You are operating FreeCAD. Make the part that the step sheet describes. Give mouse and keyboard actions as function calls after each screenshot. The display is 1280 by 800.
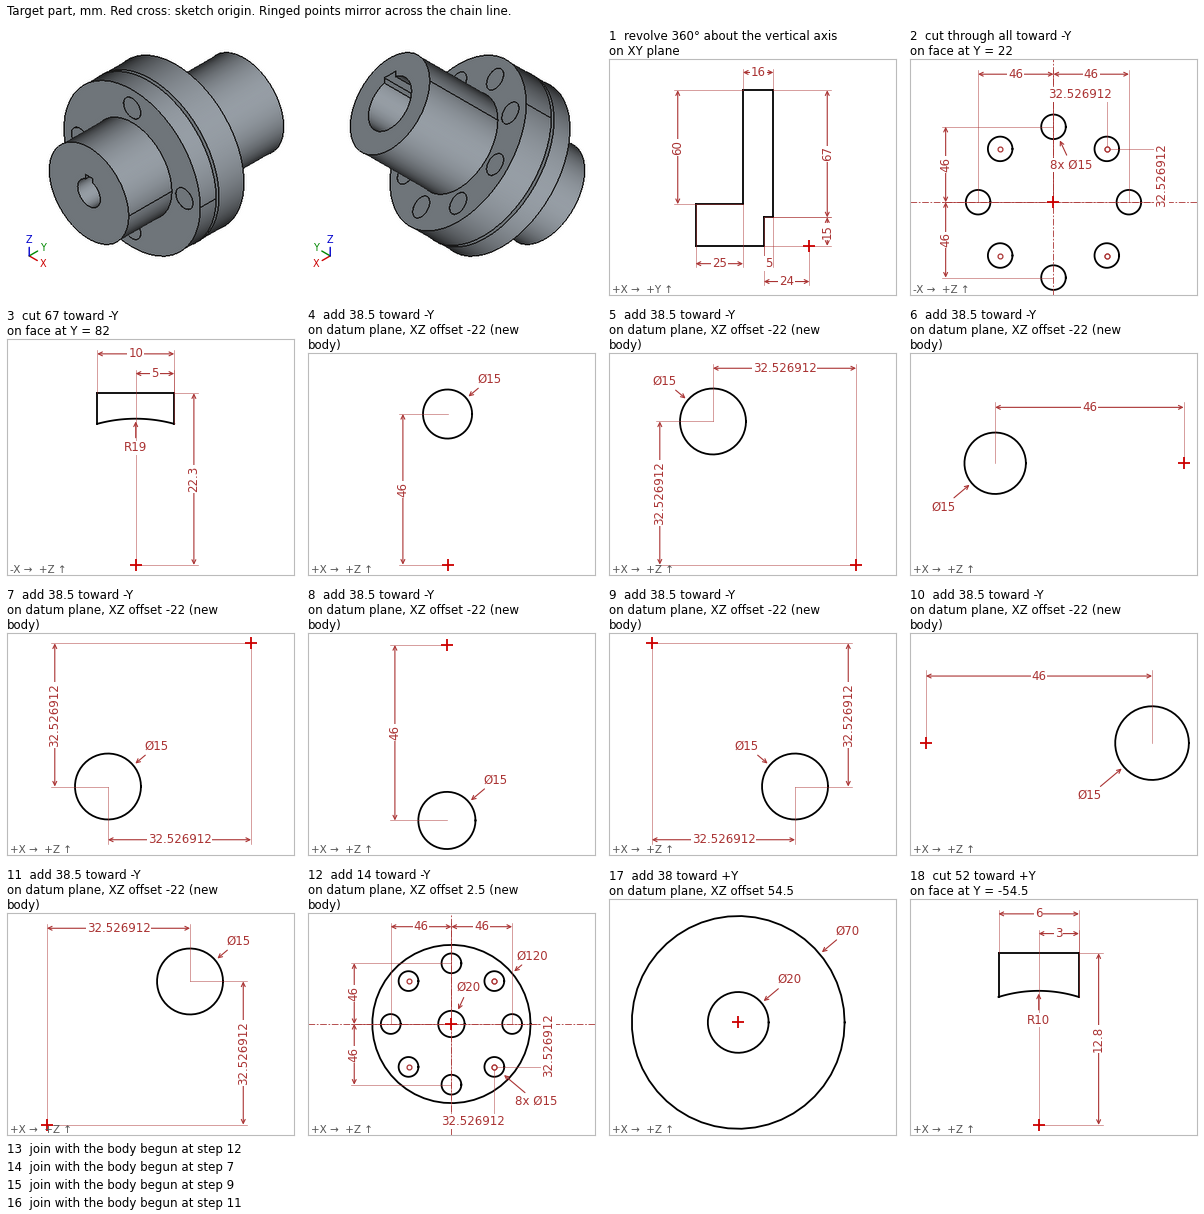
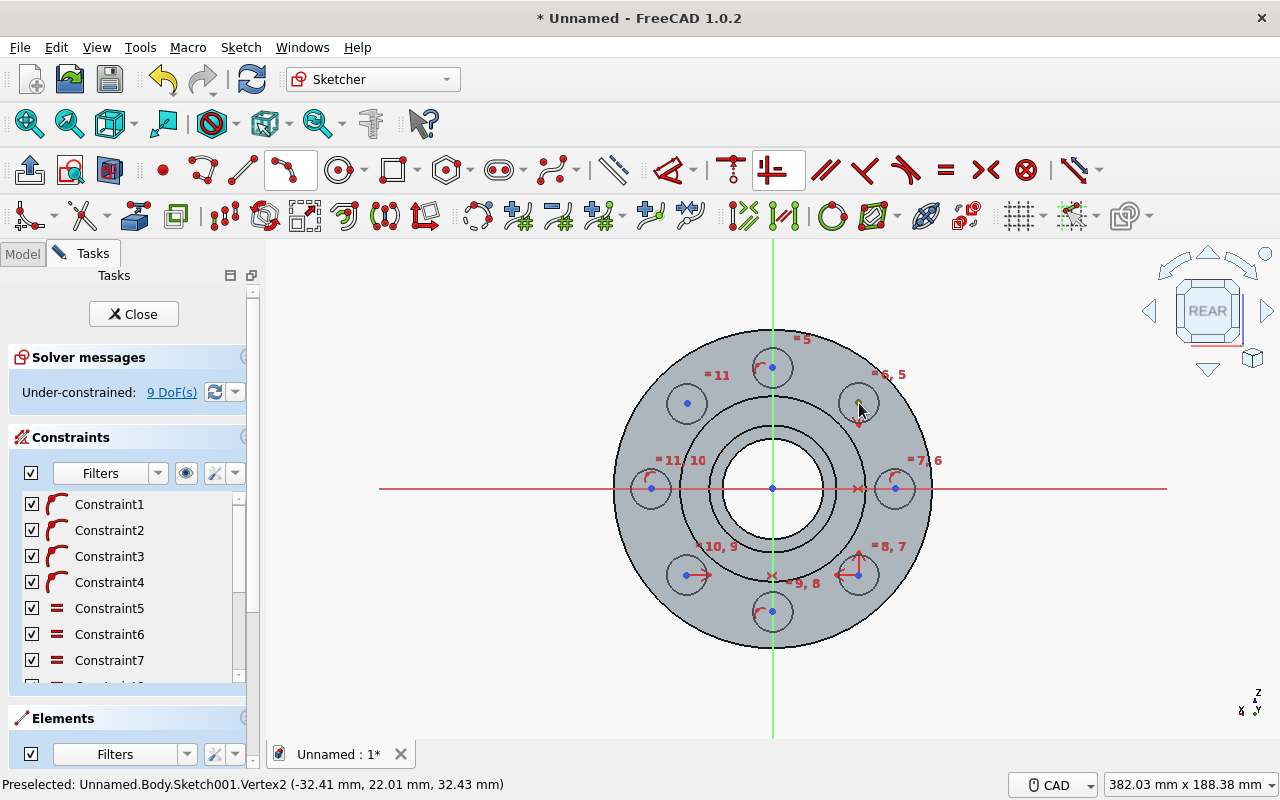
click(687, 404)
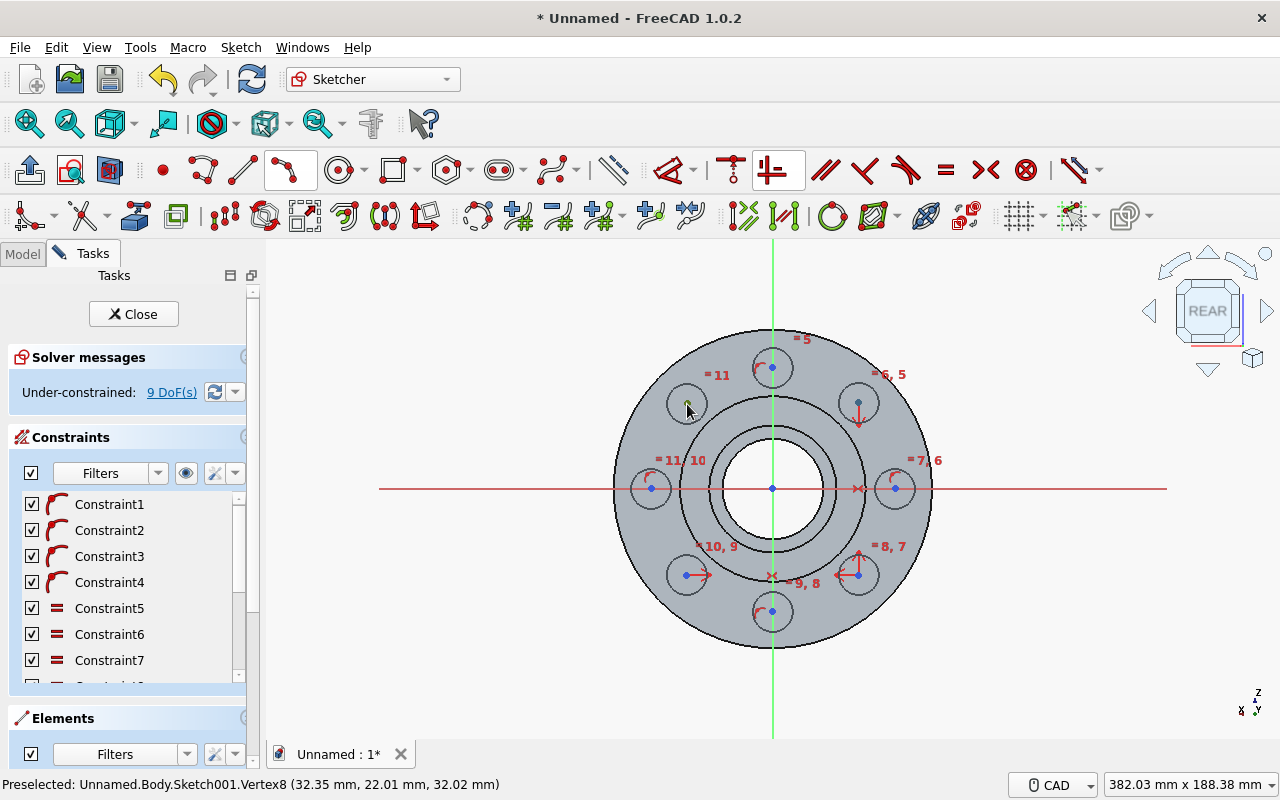
click(773, 679)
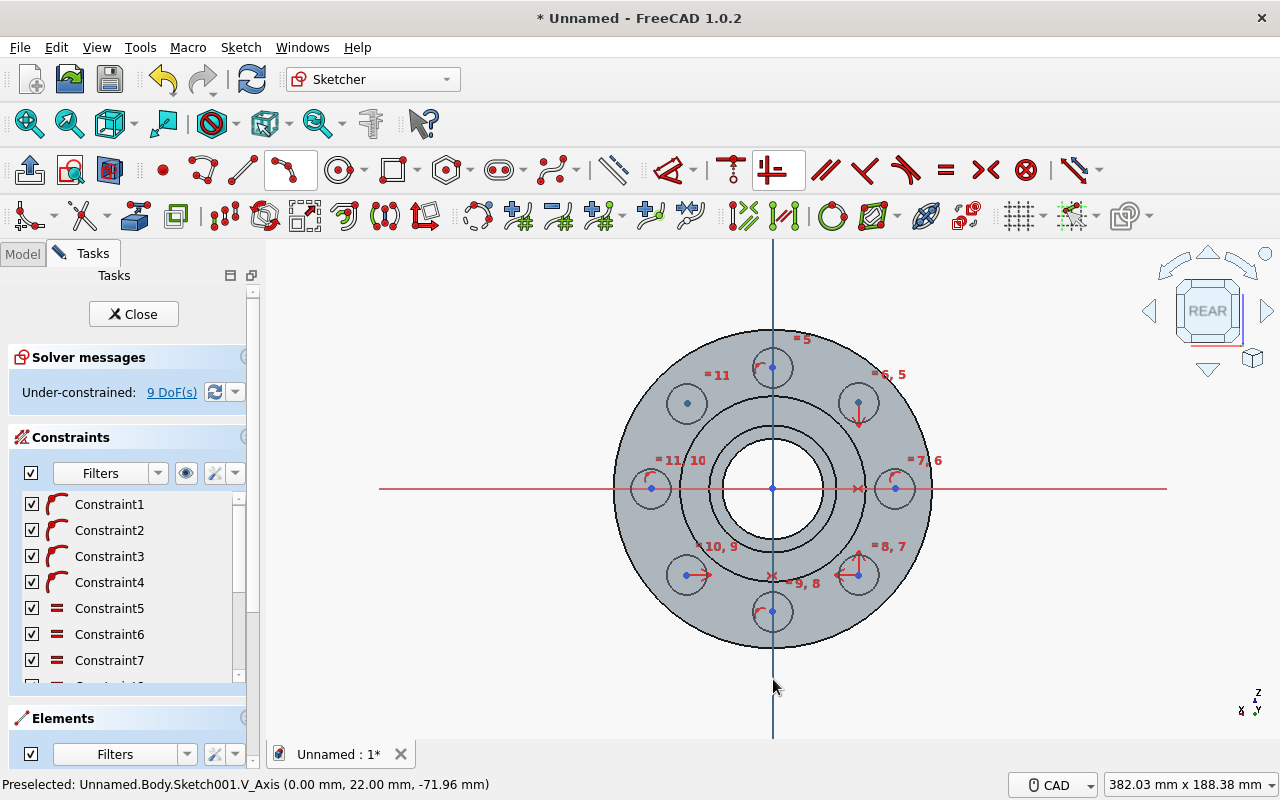
click(986, 170)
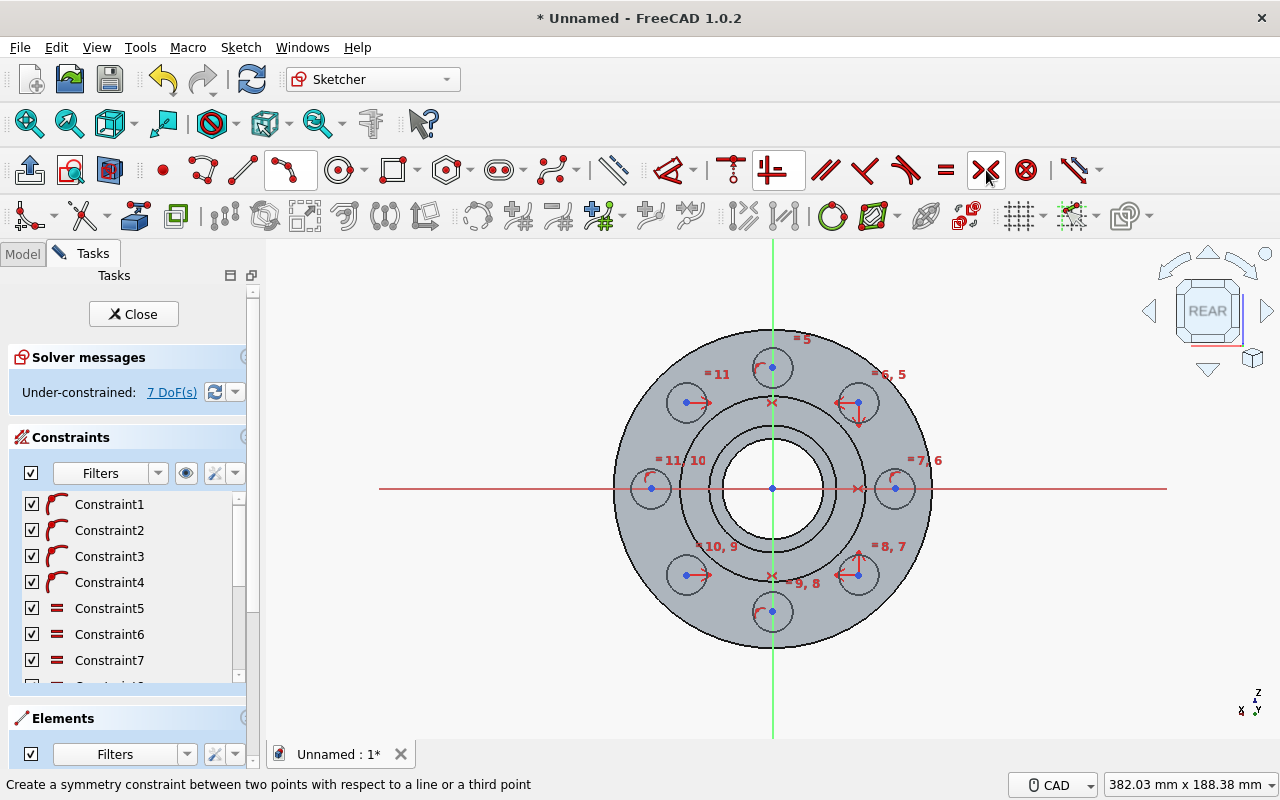
click(668, 170)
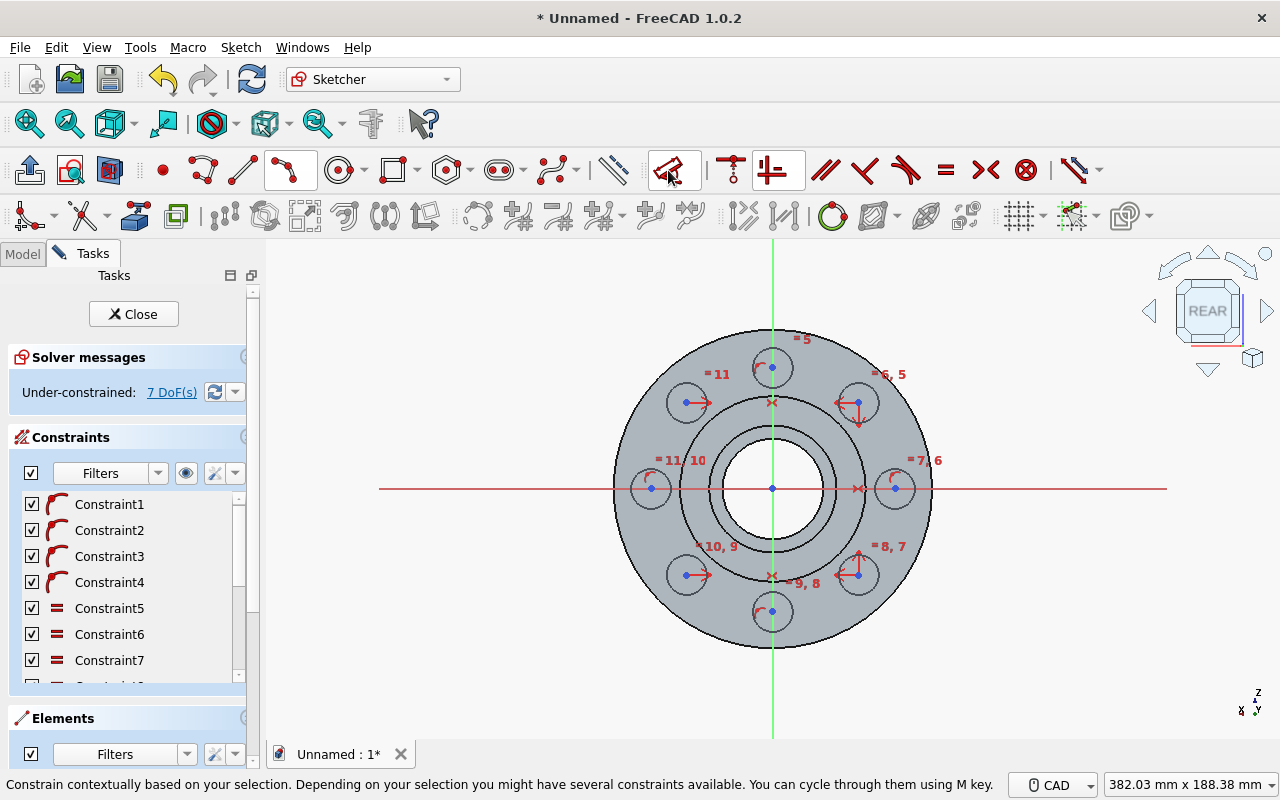
click(787, 354)
click(810, 331)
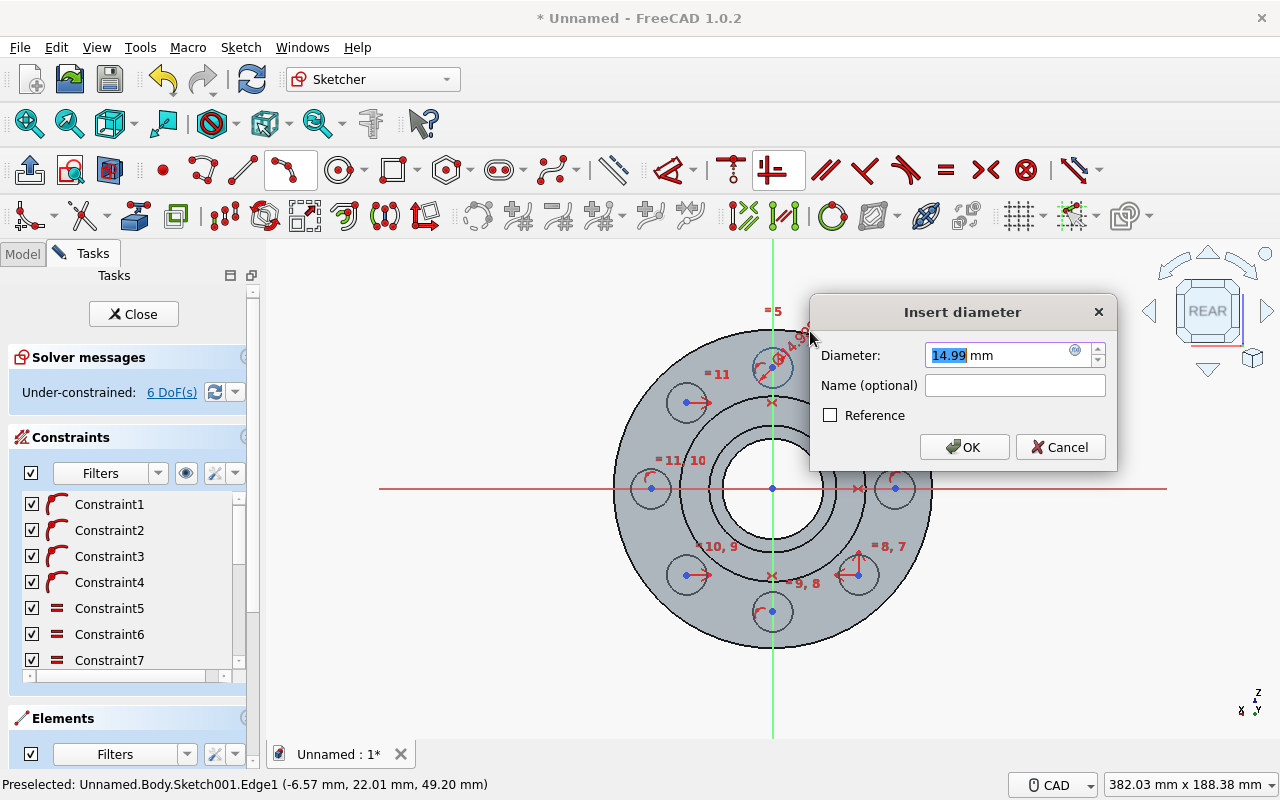
text(15)
key(Return)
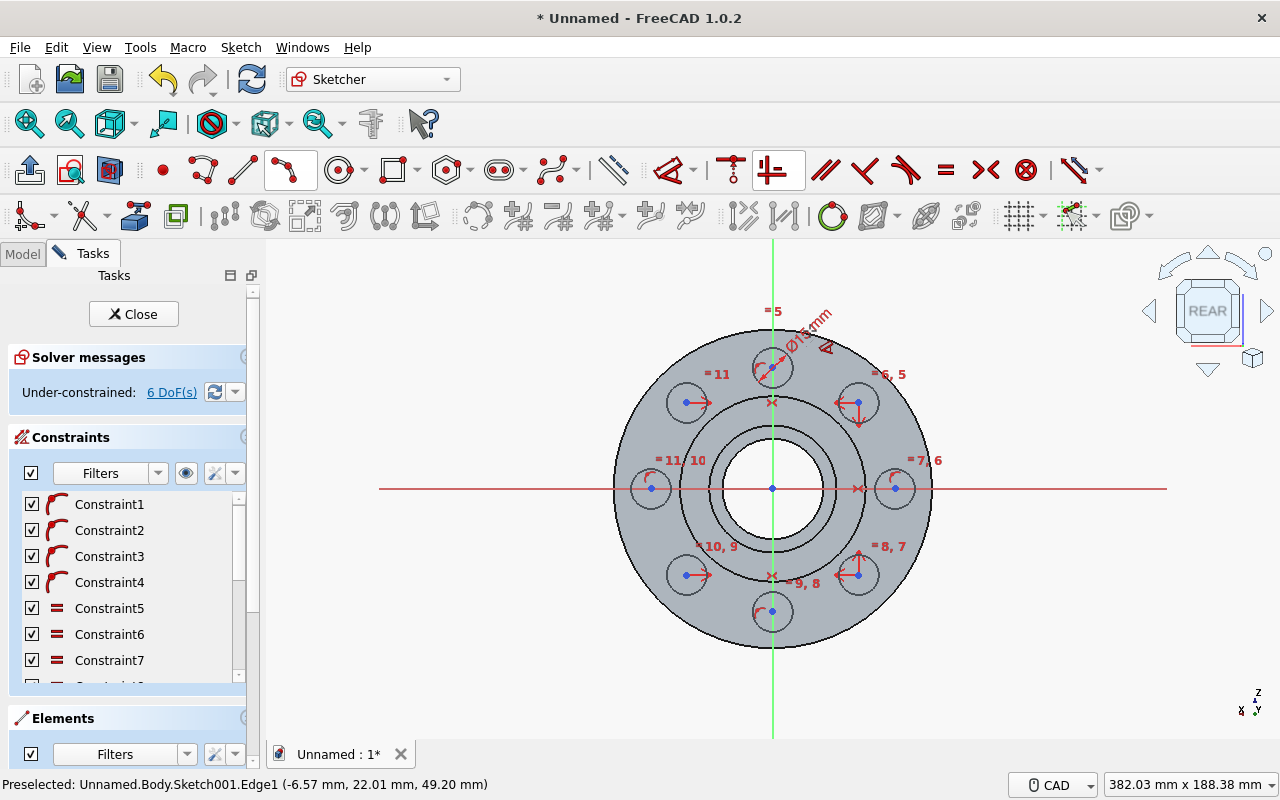
click(773, 368)
click(807, 428)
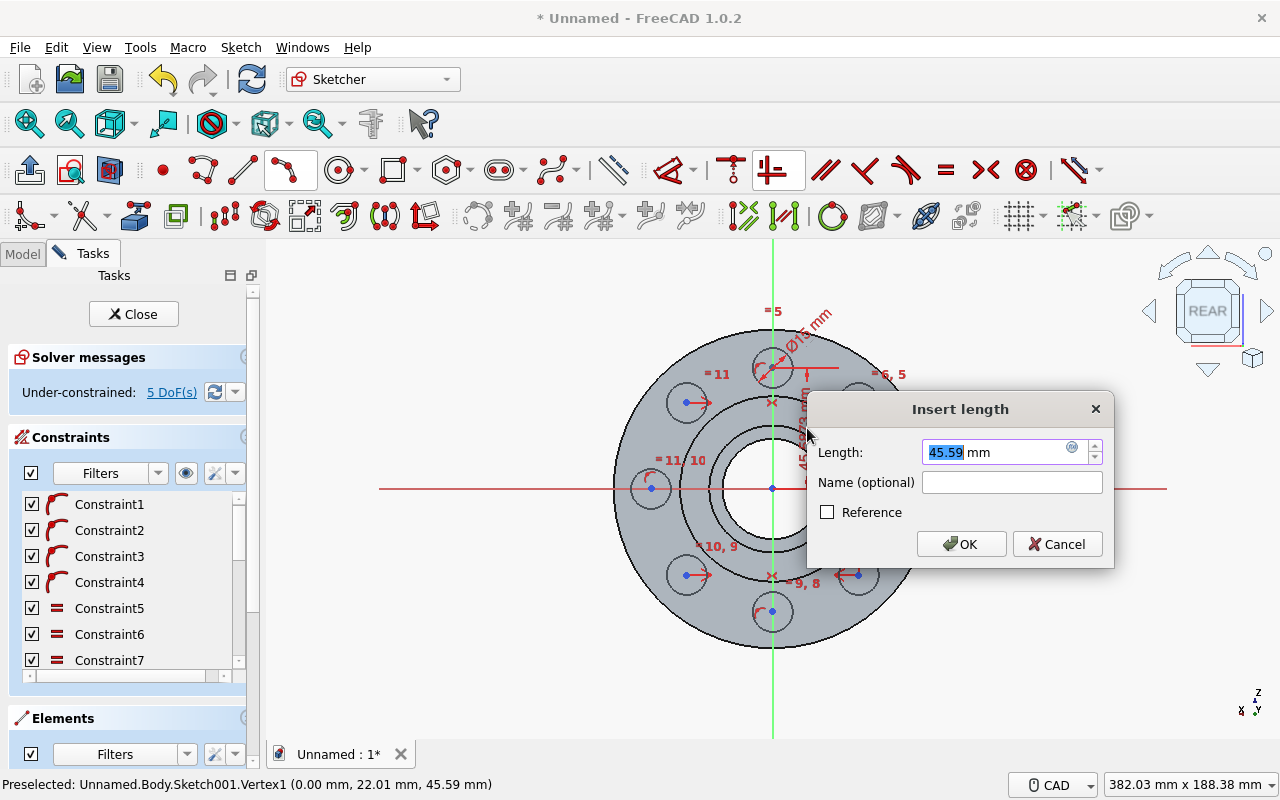
text(46)
key(Return)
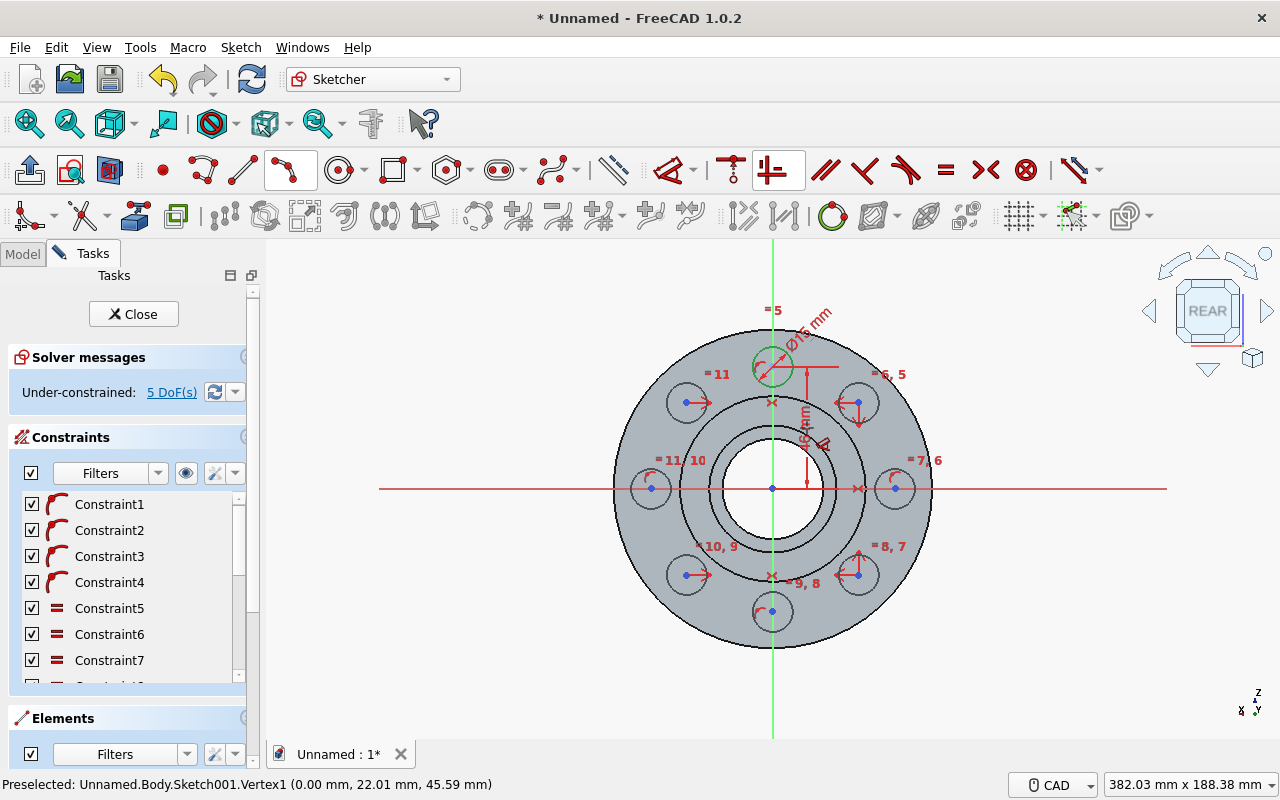
click(895, 489)
click(834, 523)